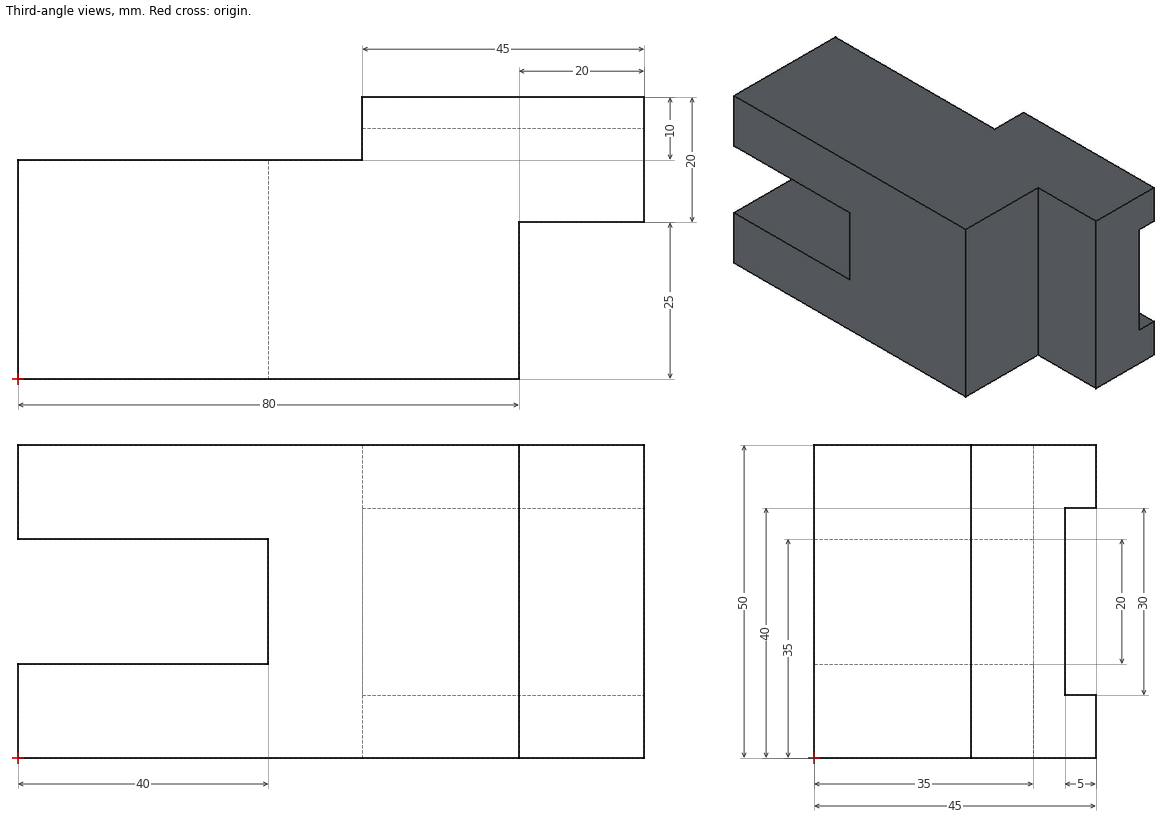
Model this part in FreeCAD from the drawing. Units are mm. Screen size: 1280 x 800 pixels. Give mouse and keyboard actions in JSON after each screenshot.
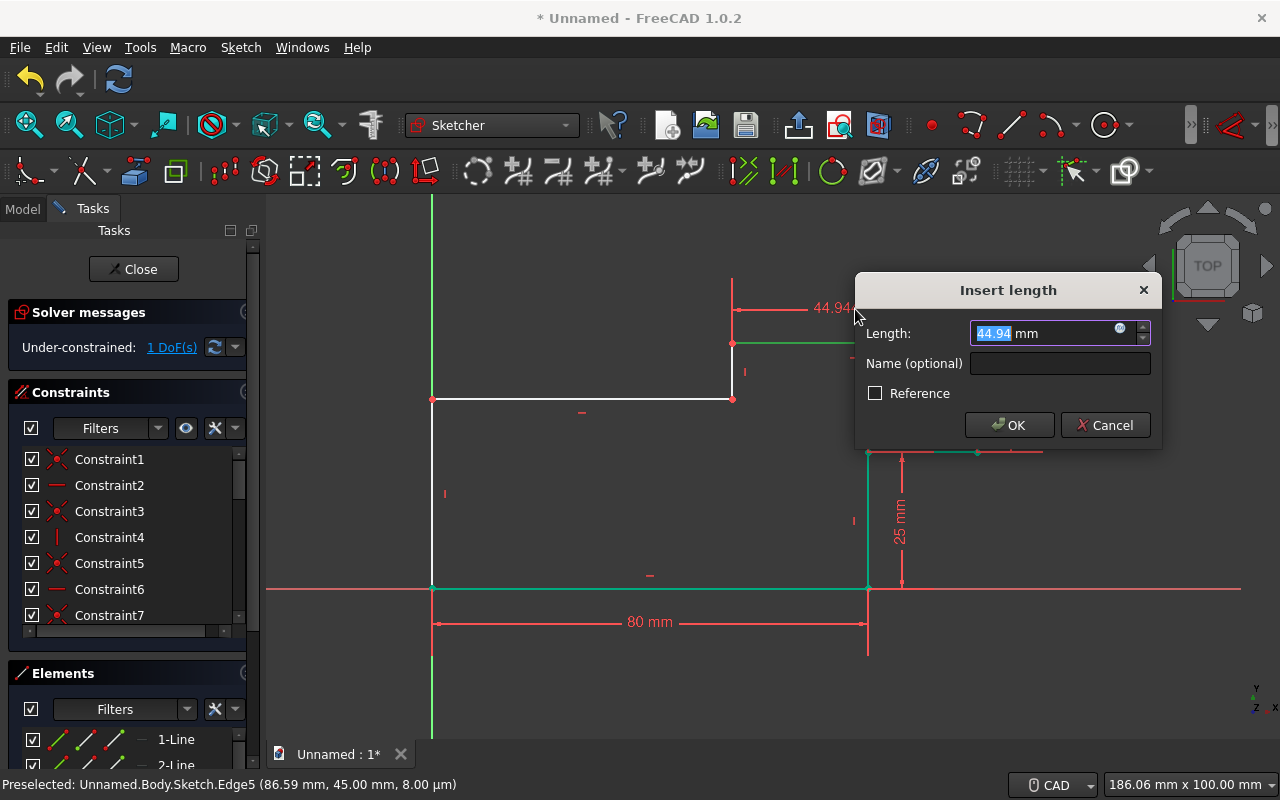
{"action": "type", "text": "45"}
{"action": "key", "text": "Return"}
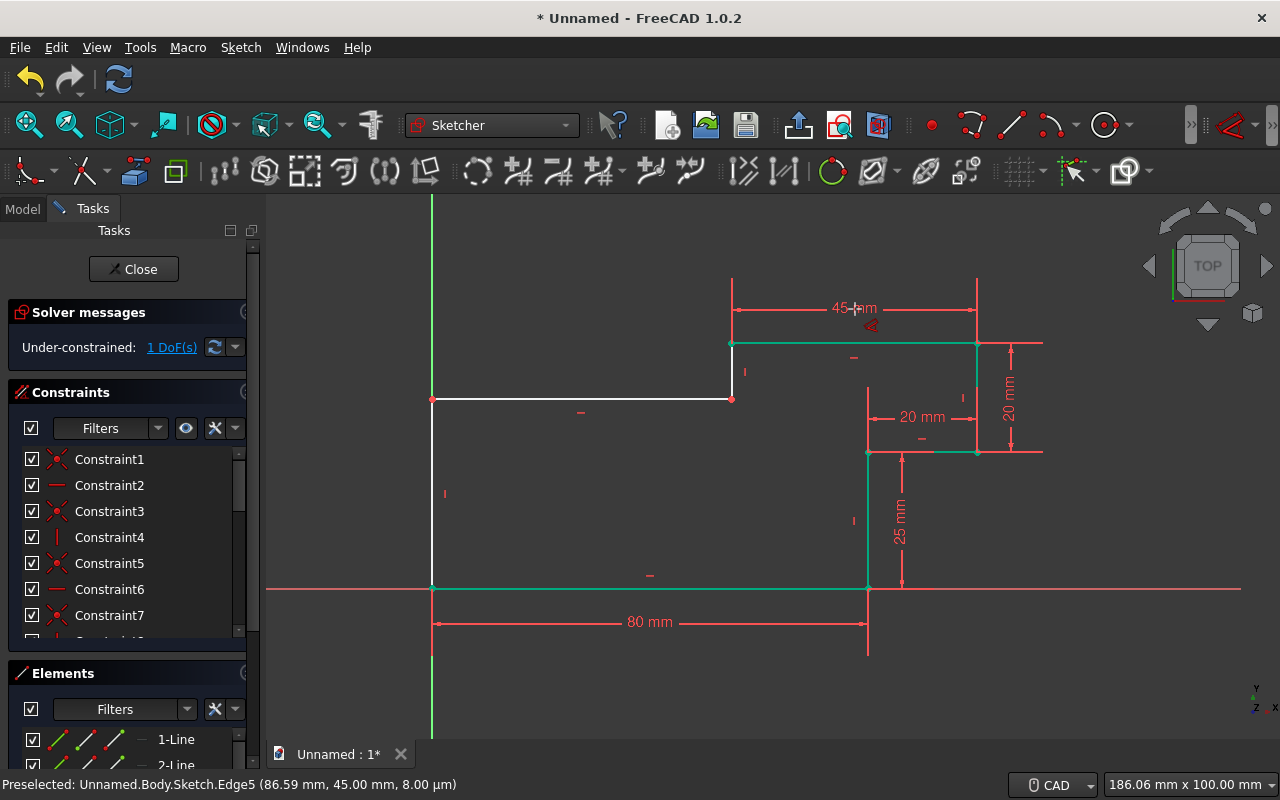
{"action": "left_click", "coordinate": [732, 360]}
{"action": "left_click", "coordinate": [766, 371]}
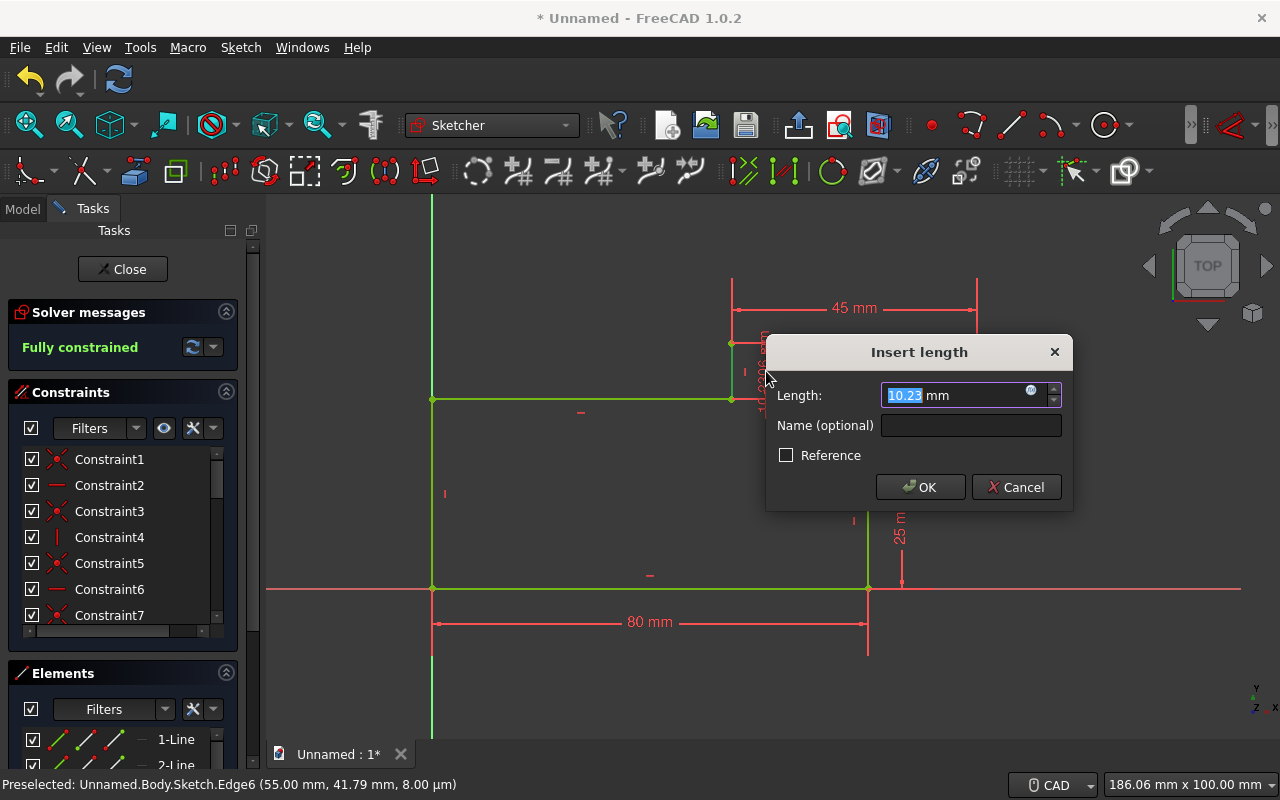
{"action": "type", "text": "10"}
{"action": "key", "text": "Return"}
{"action": "key", "text": "Escape"}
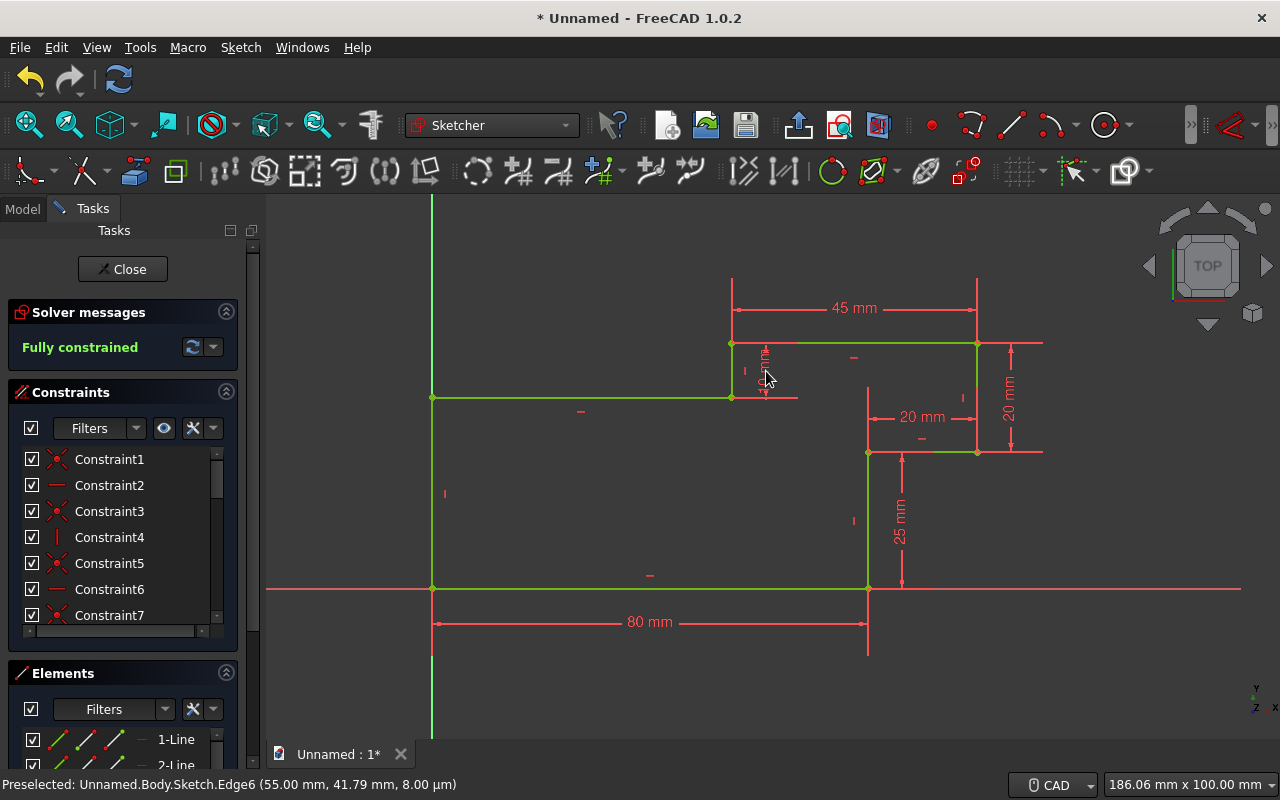
{"action": "left_click", "coordinate": [123, 269]}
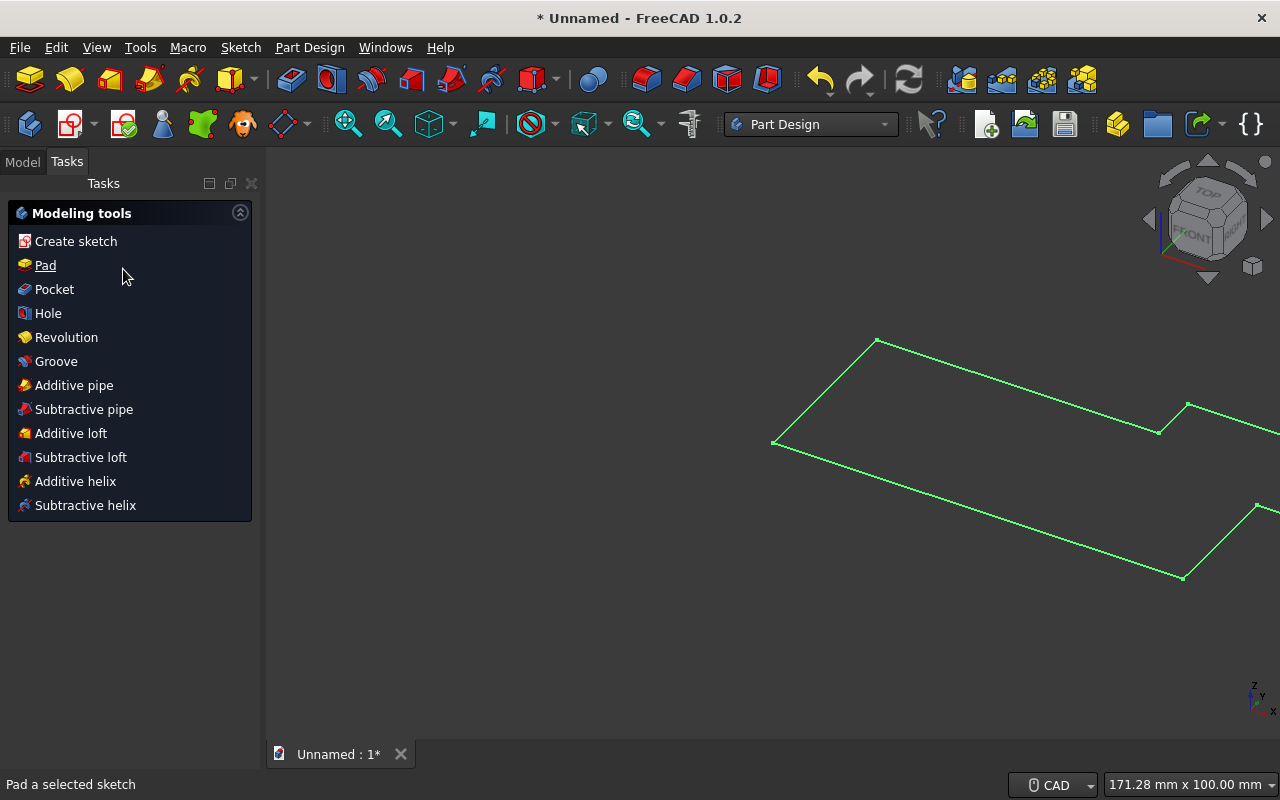
{"action": "left_click", "coordinate": [30, 80]}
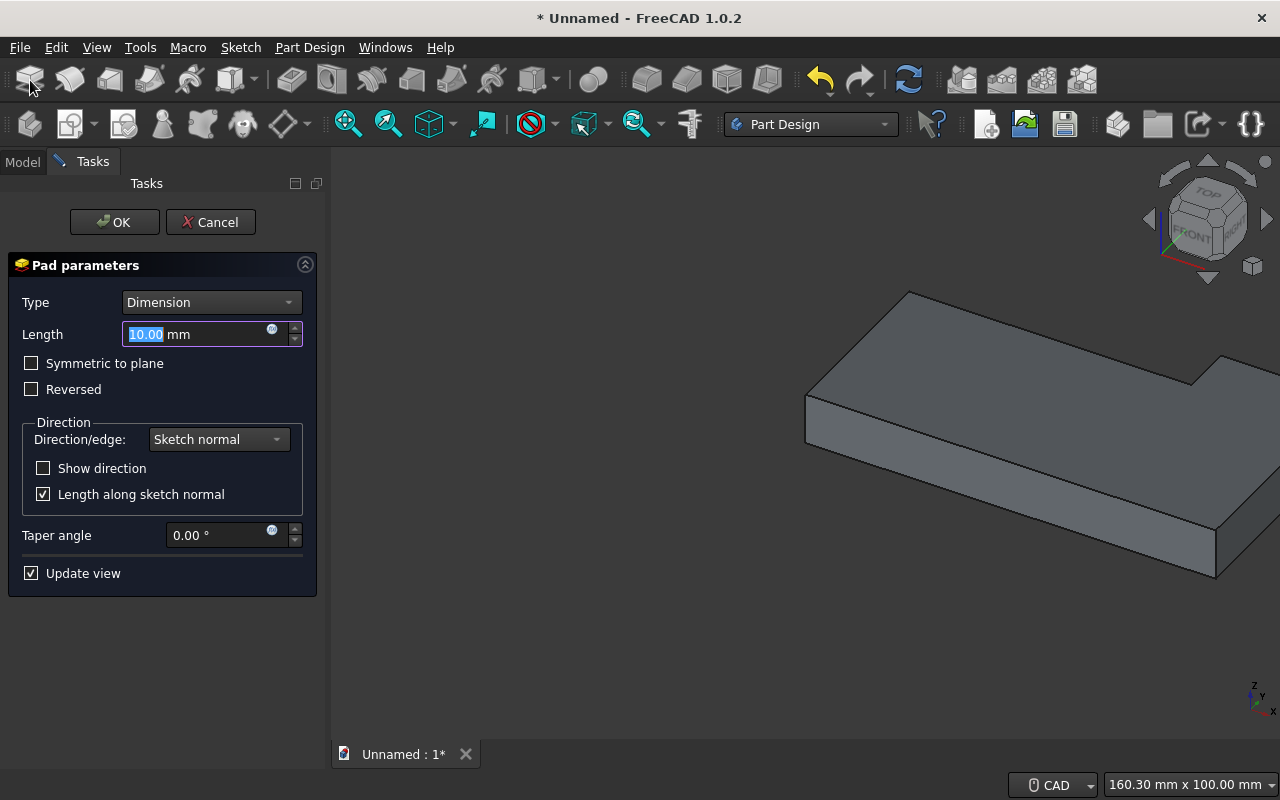
{"action": "type", "text": "50"}
{"action": "key", "text": "Tab"}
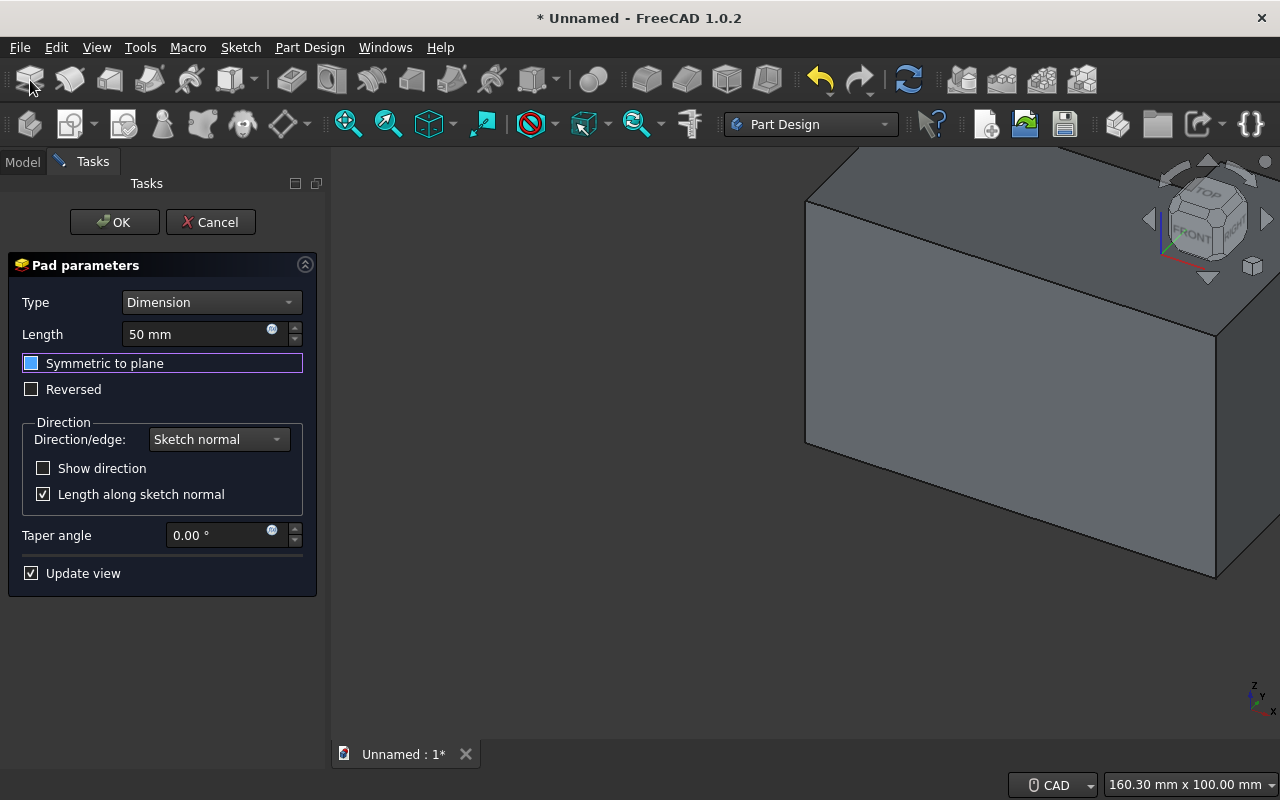
{"action": "left_click", "coordinate": [115, 222]}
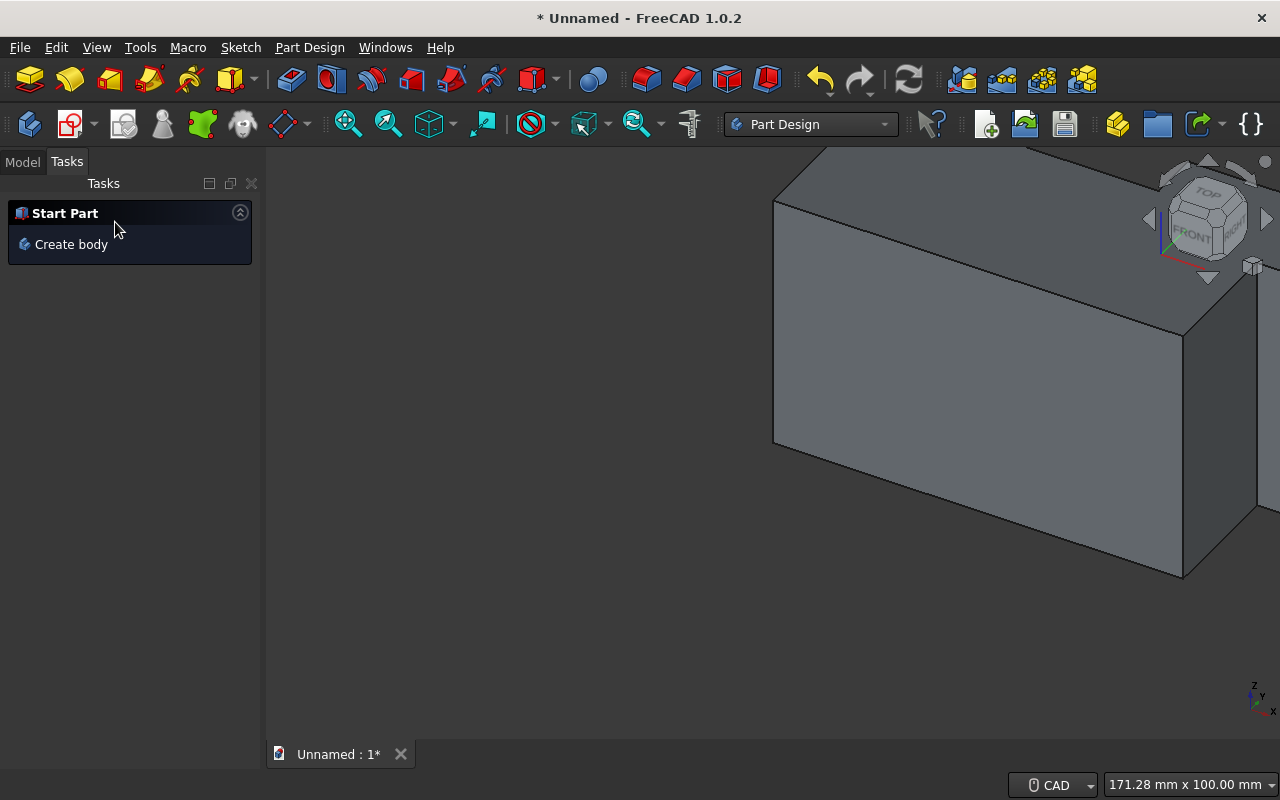
{"action": "left_click", "coordinate": [350, 124]}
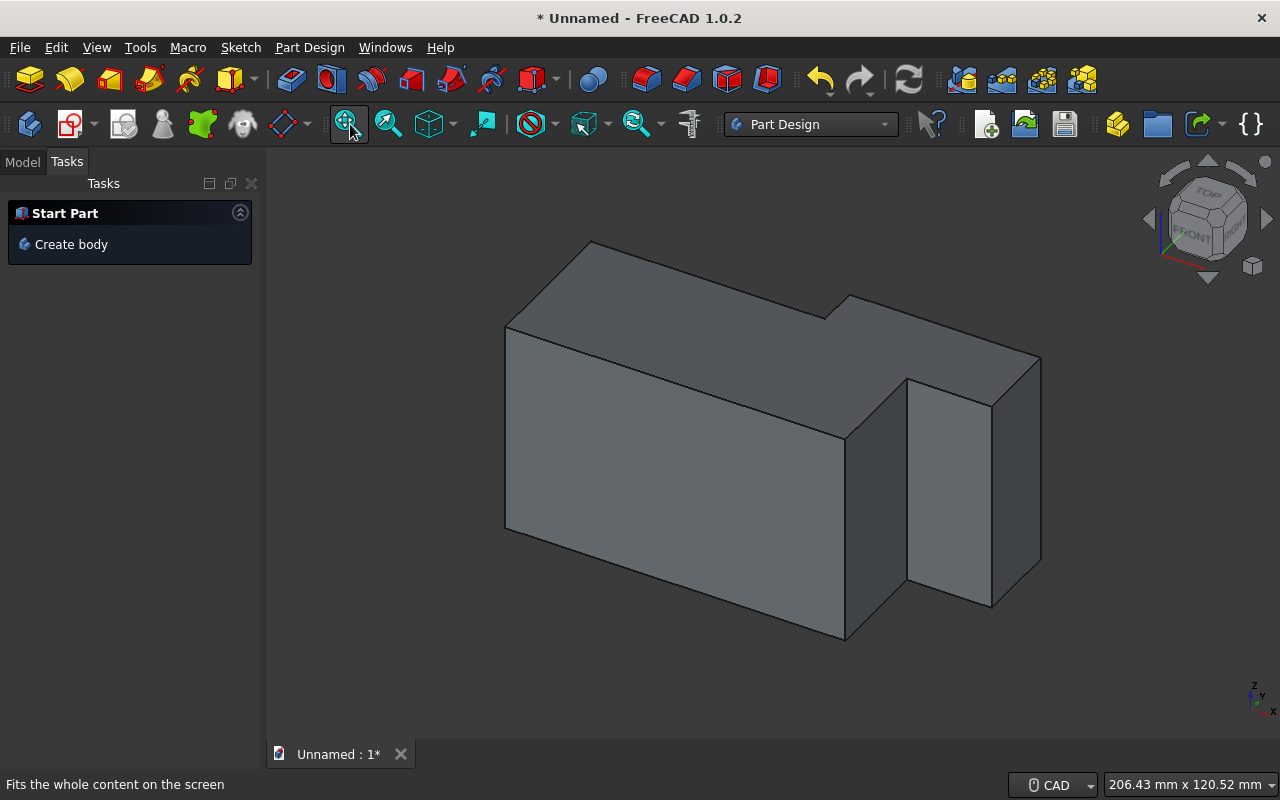
{"action": "left_click", "coordinate": [70, 124]}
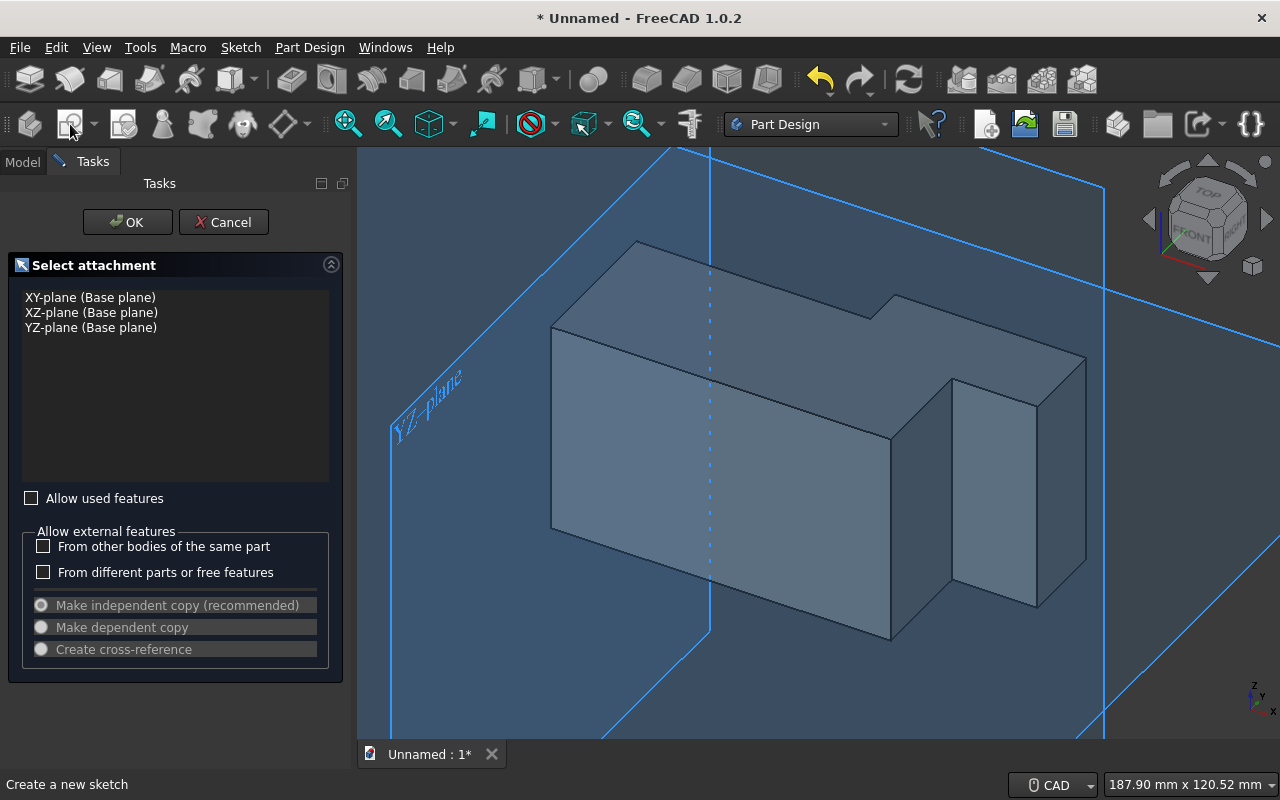
{"action": "left_click", "coordinate": [82, 328]}